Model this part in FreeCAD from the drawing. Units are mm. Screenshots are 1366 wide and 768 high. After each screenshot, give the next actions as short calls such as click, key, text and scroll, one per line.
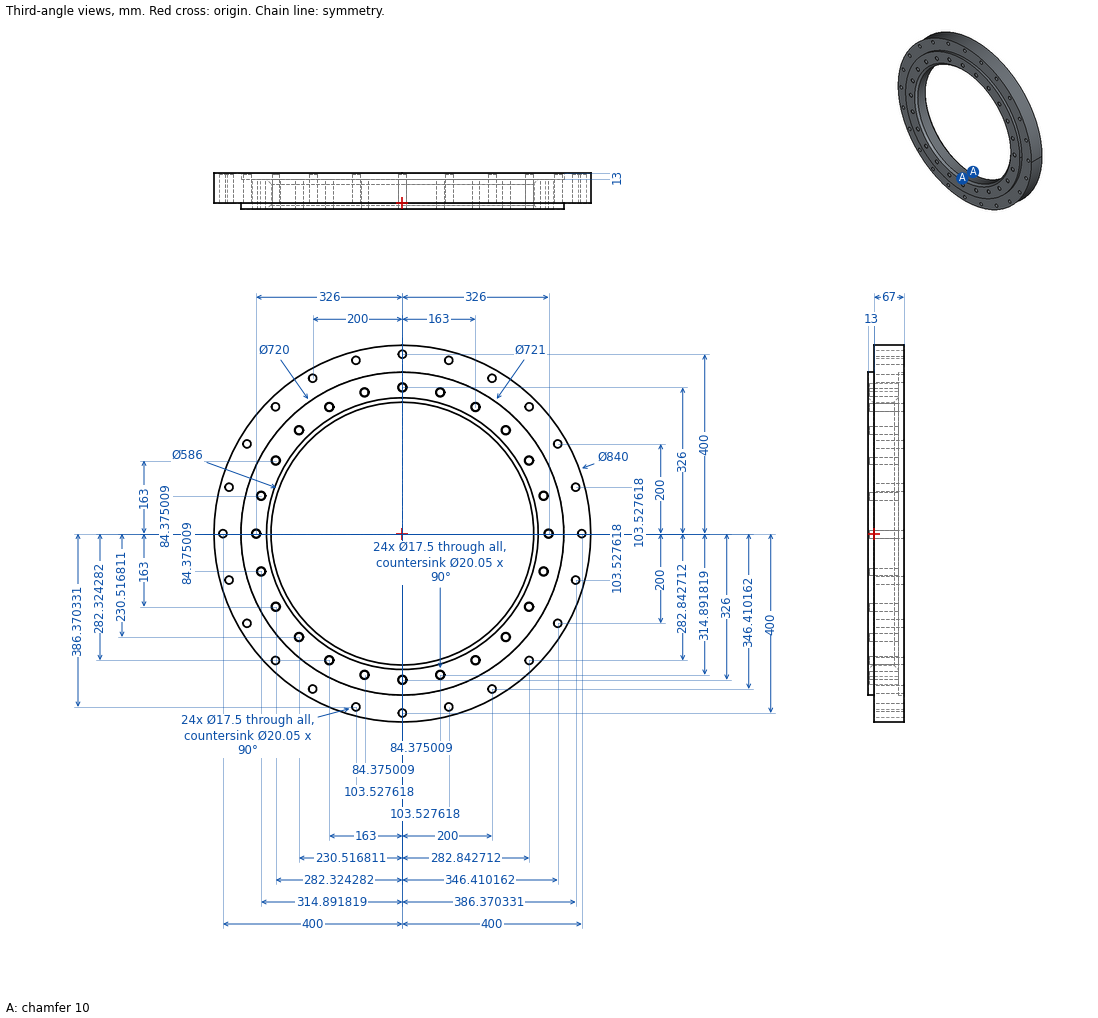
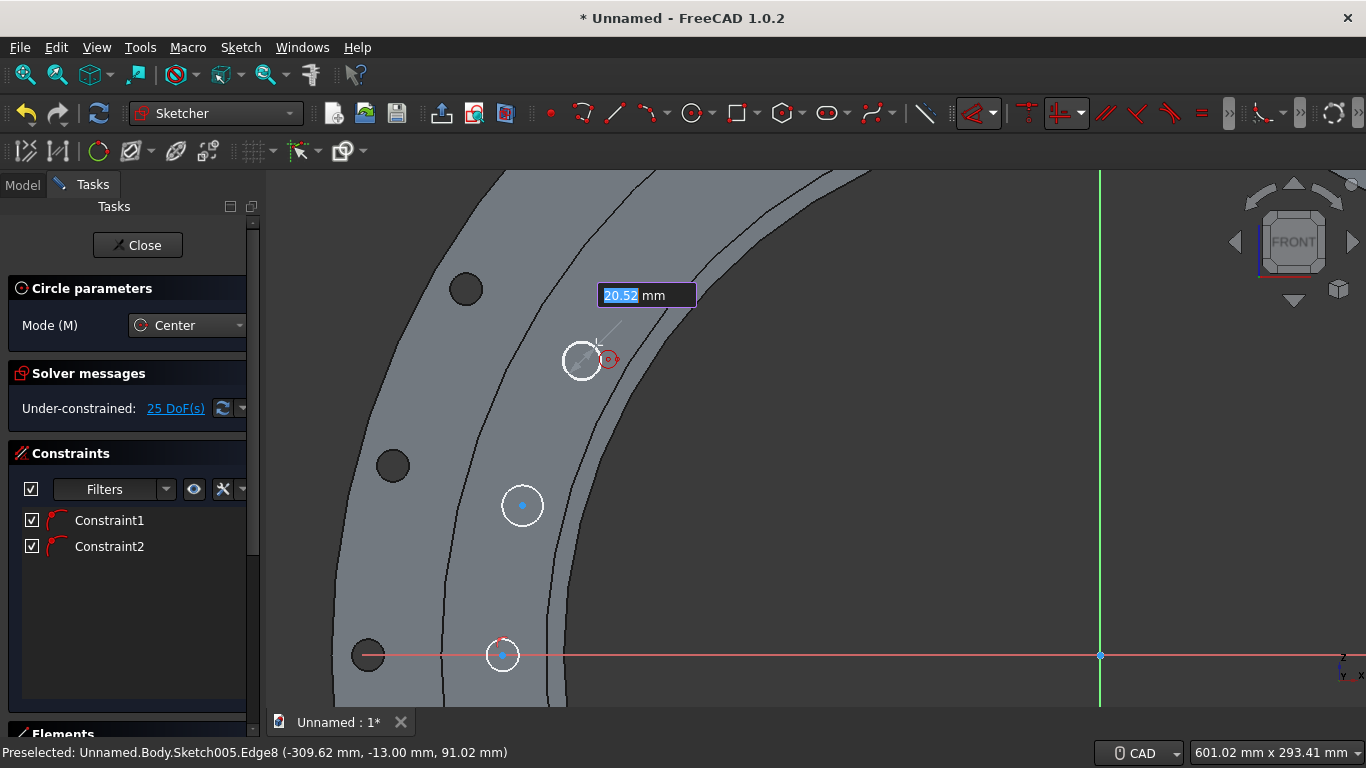
click(595, 346)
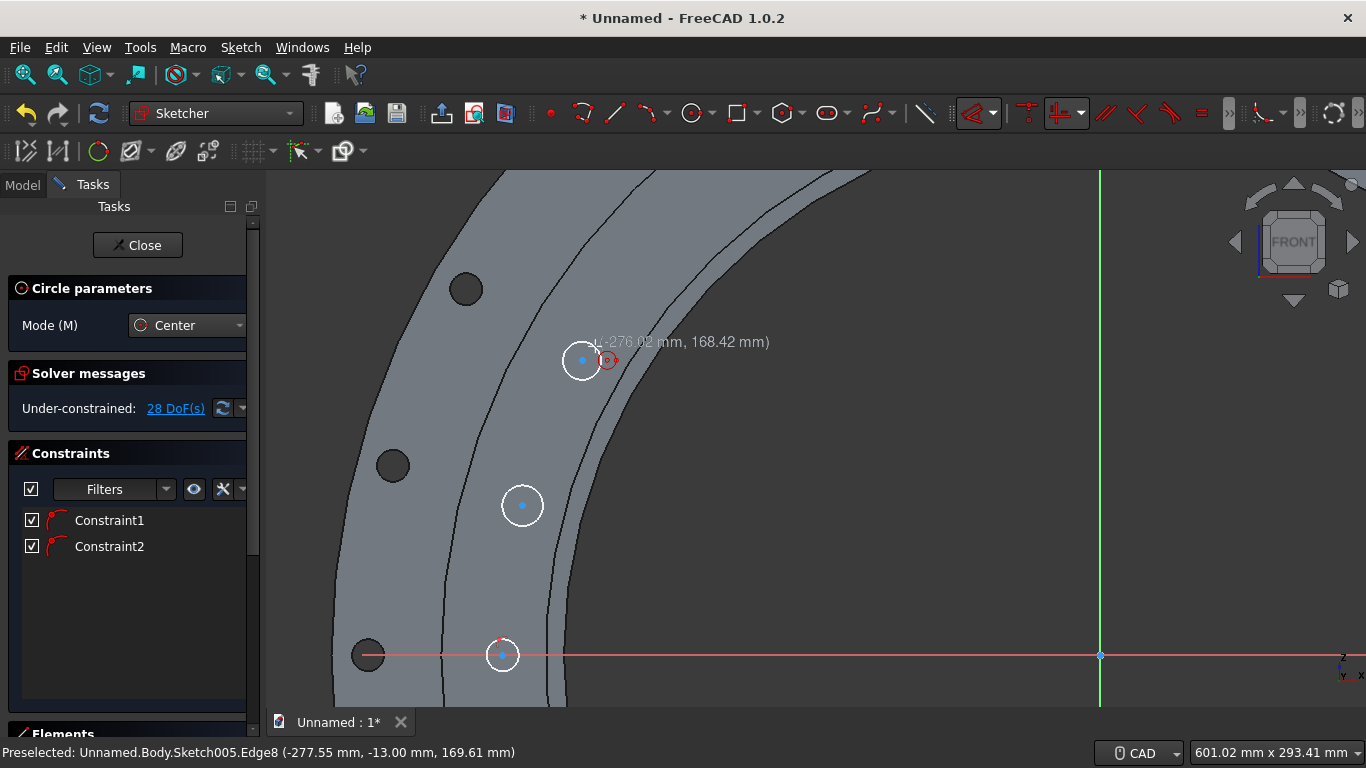
scroll(678, 233, up, 2)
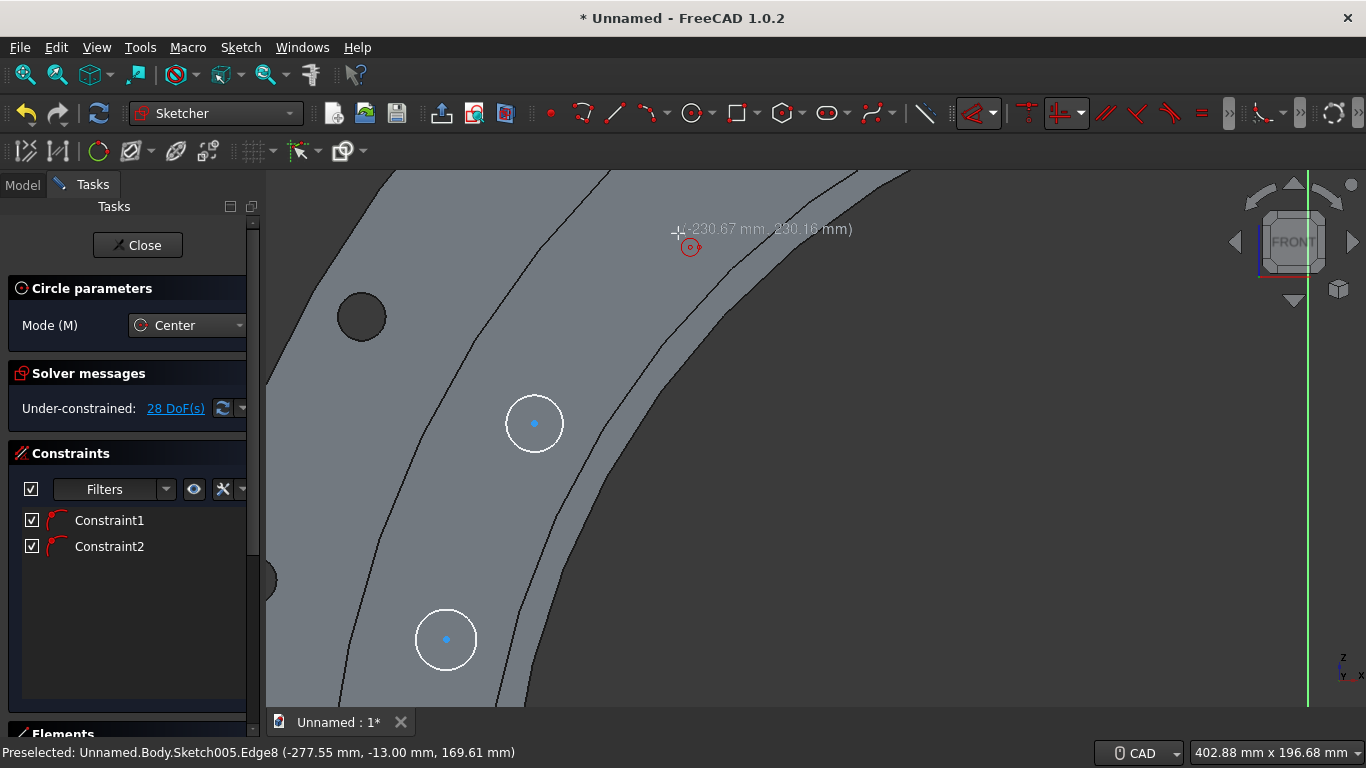
scroll(606, 331, down, 8)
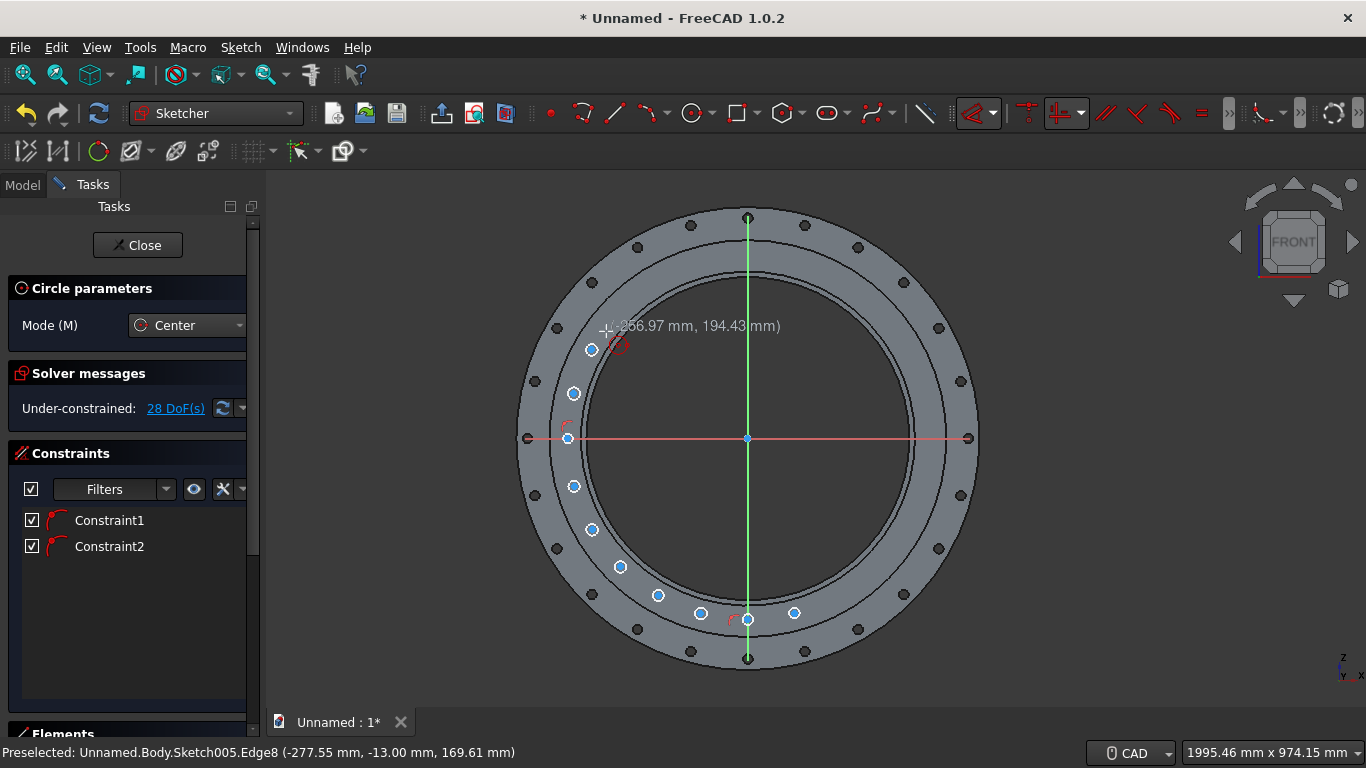
click(621, 312)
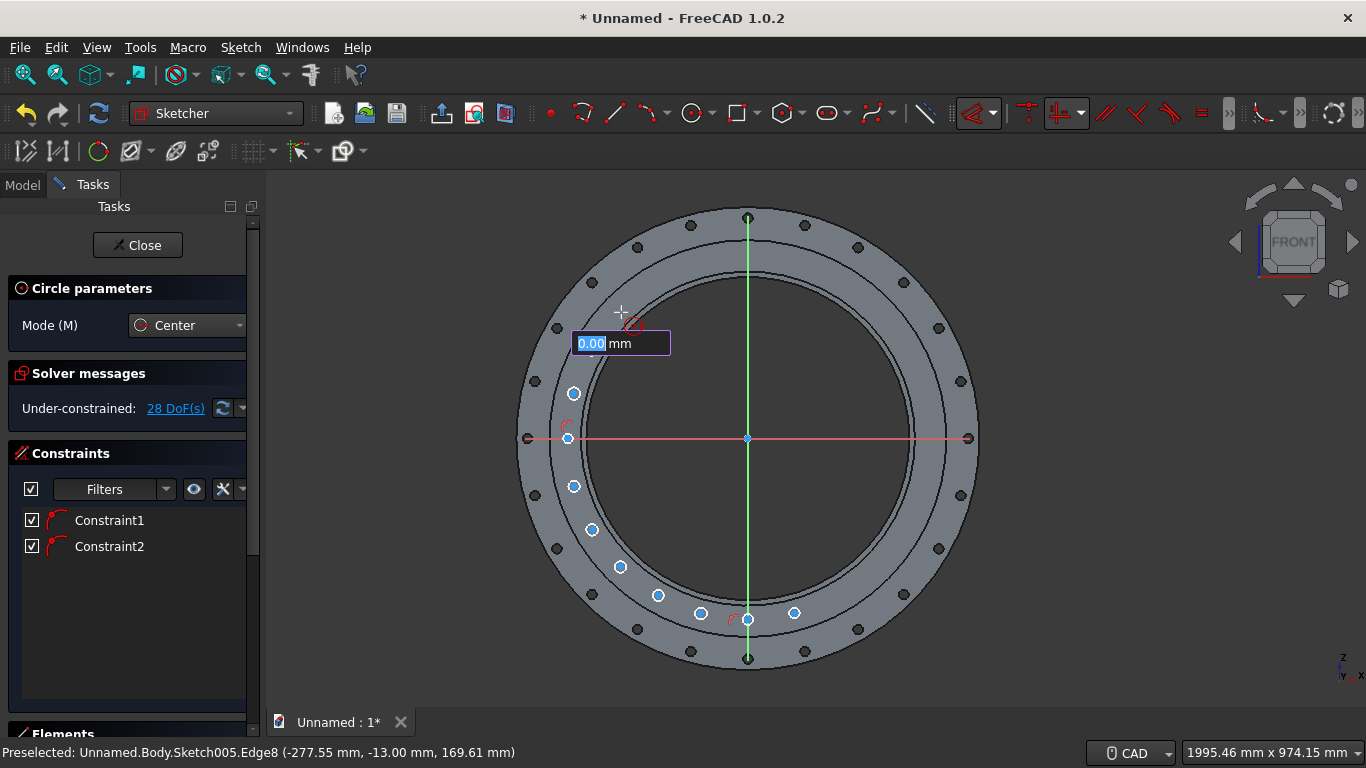
scroll(624, 308, up, 6)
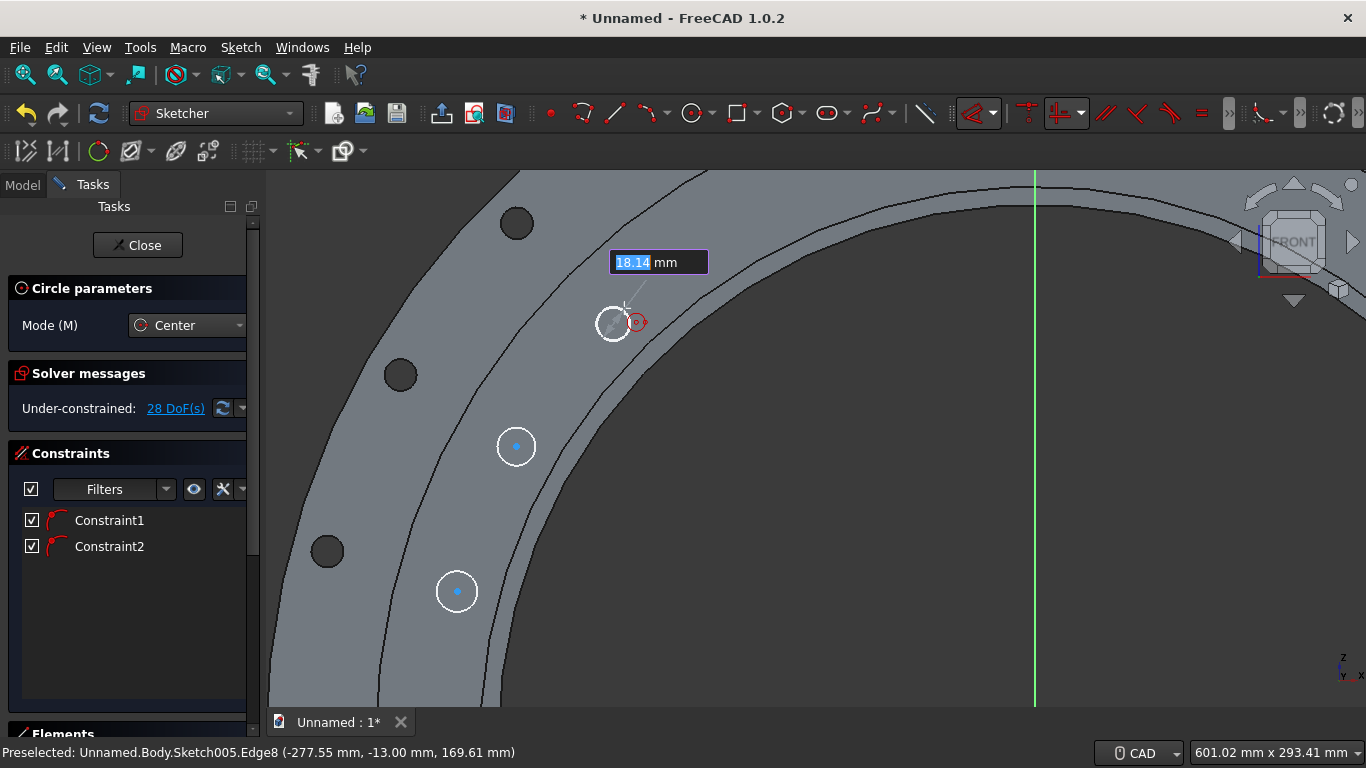
click(624, 308)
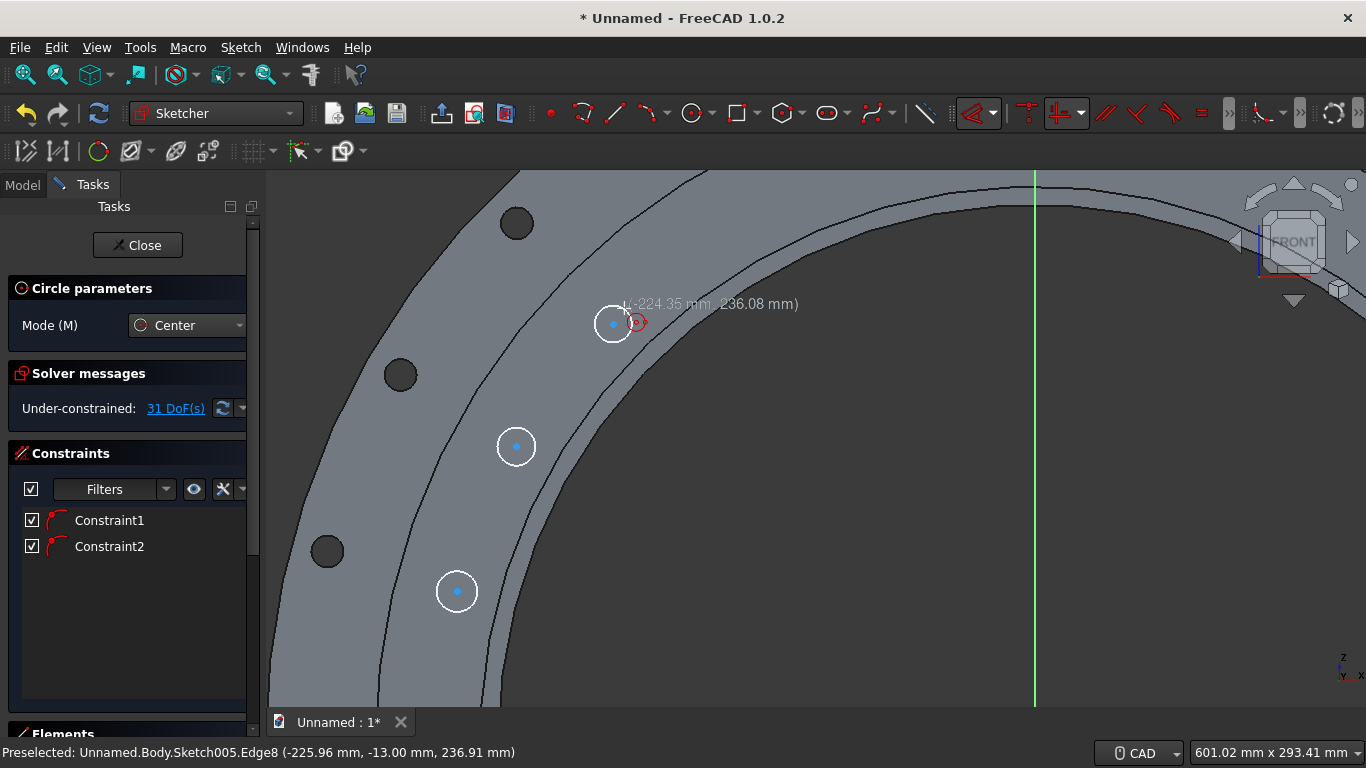
scroll(736, 224, up, 2)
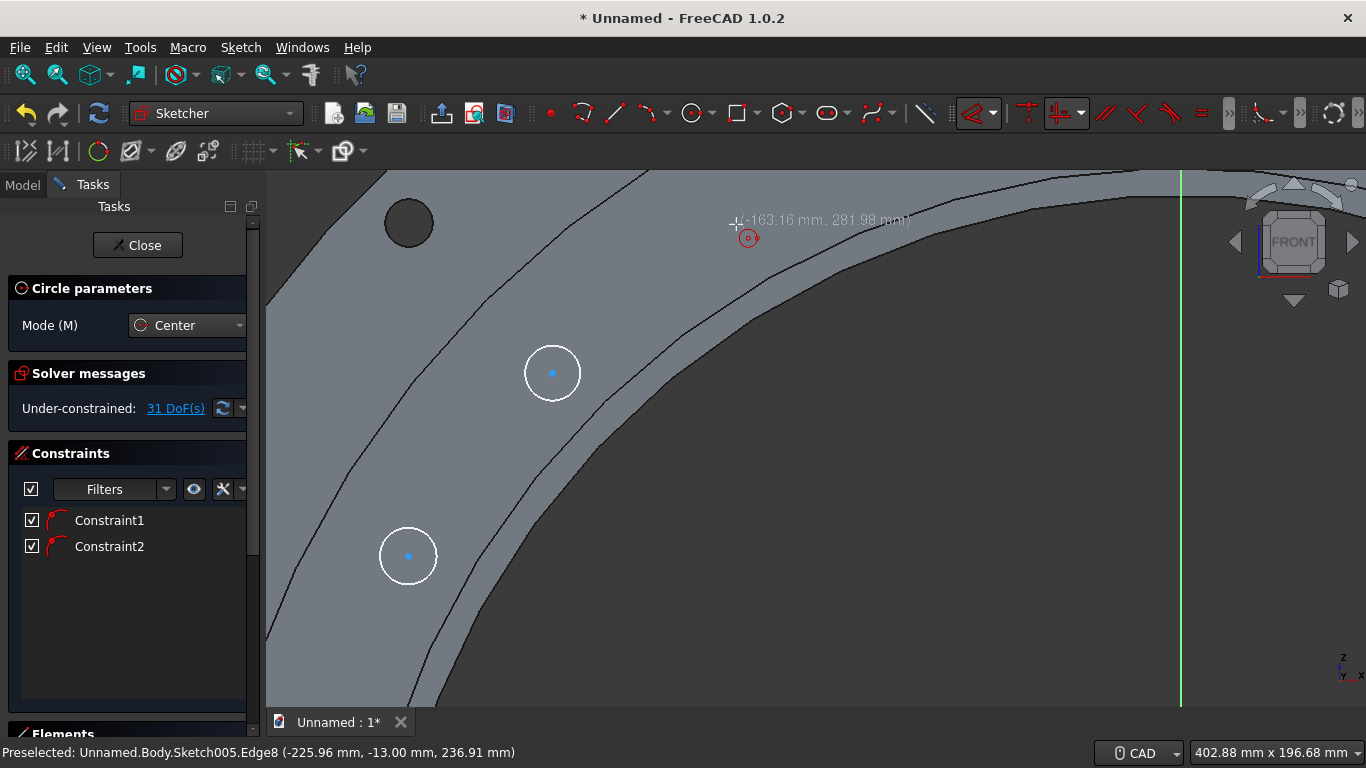
scroll(638, 298, down, 8)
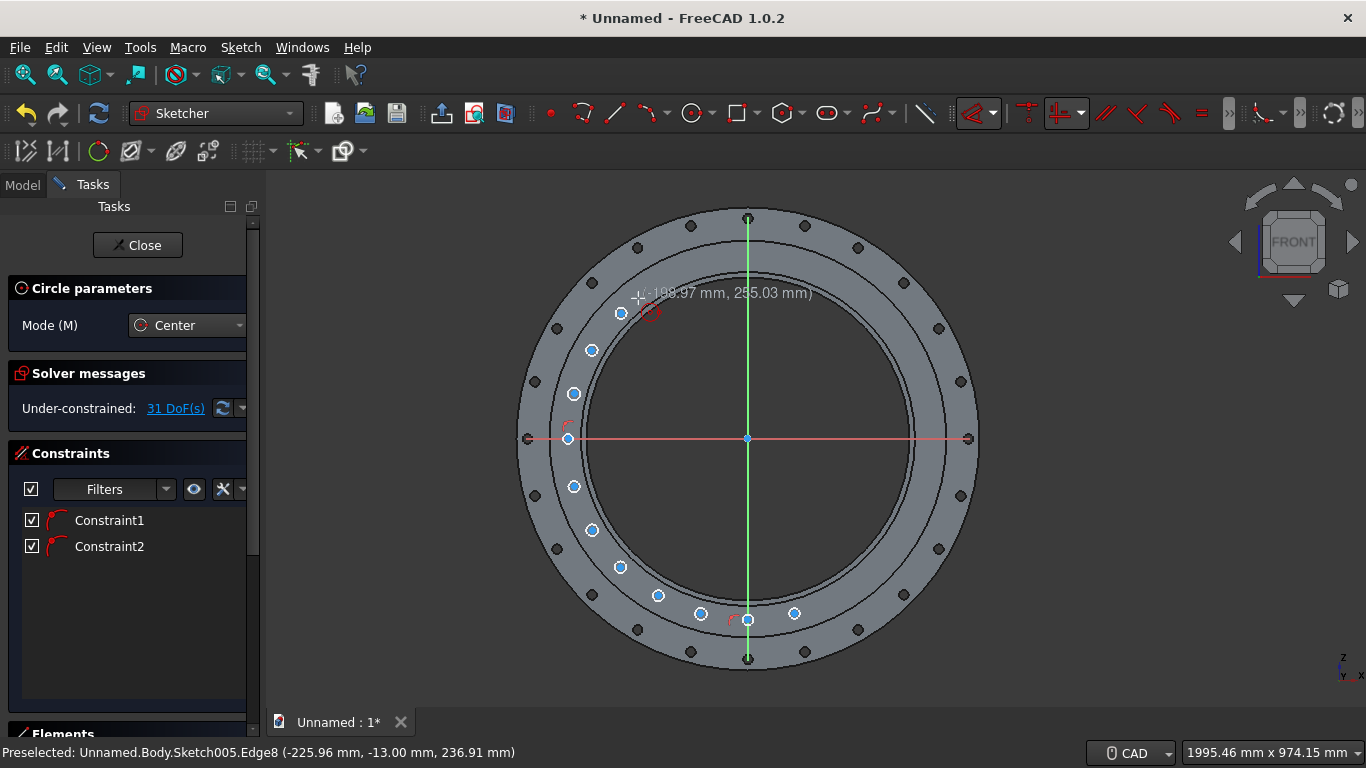
click(658, 283)